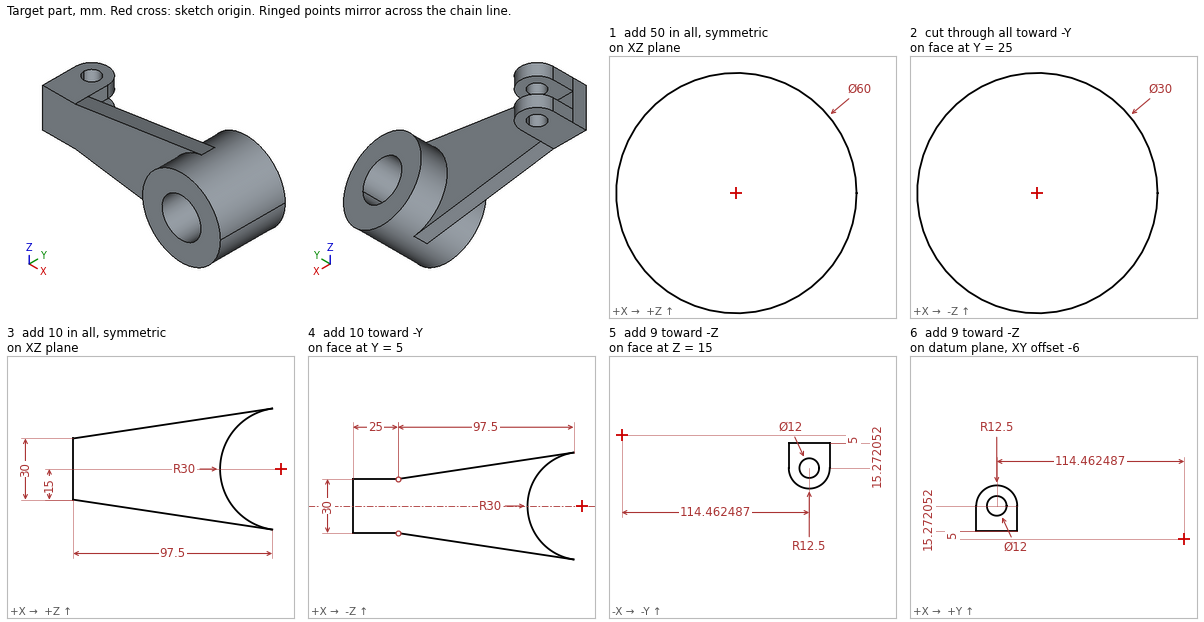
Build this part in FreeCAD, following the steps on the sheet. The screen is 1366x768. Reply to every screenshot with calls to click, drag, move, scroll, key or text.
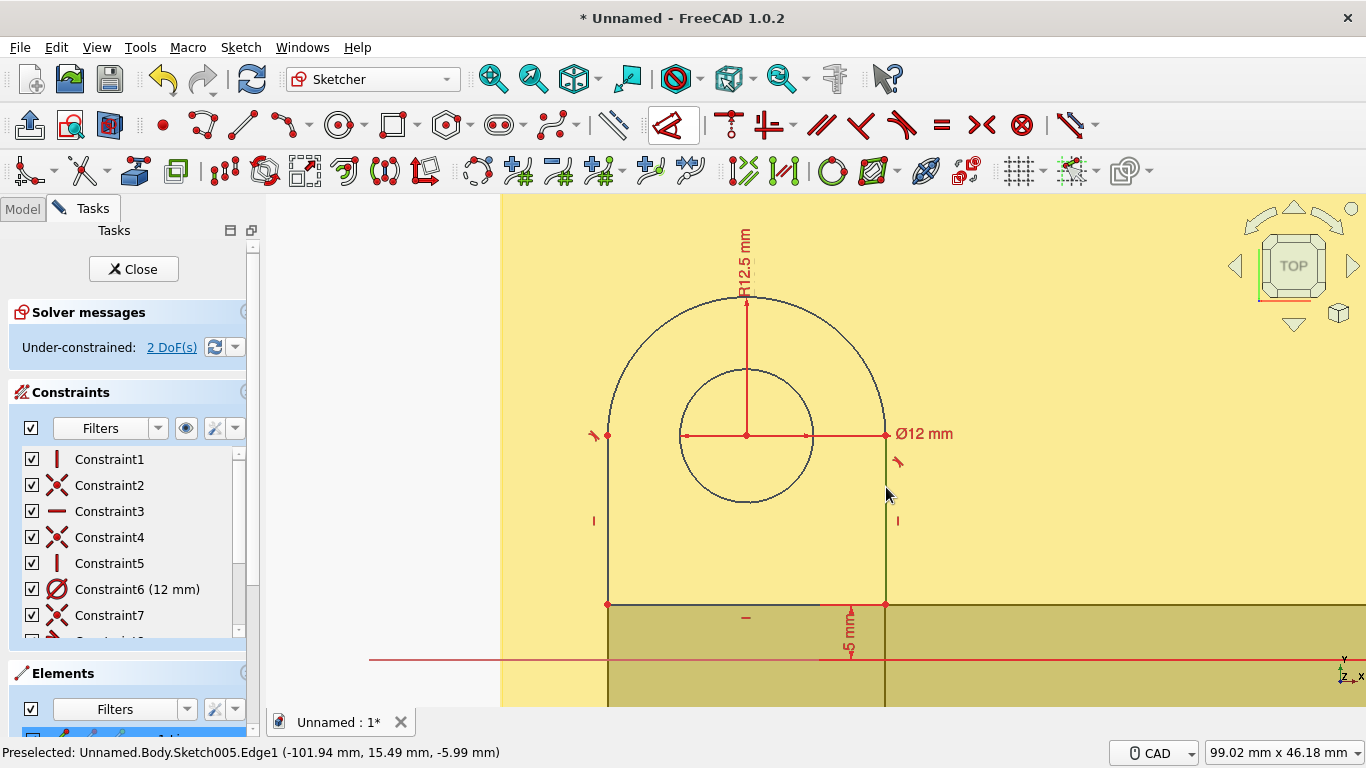
key(i)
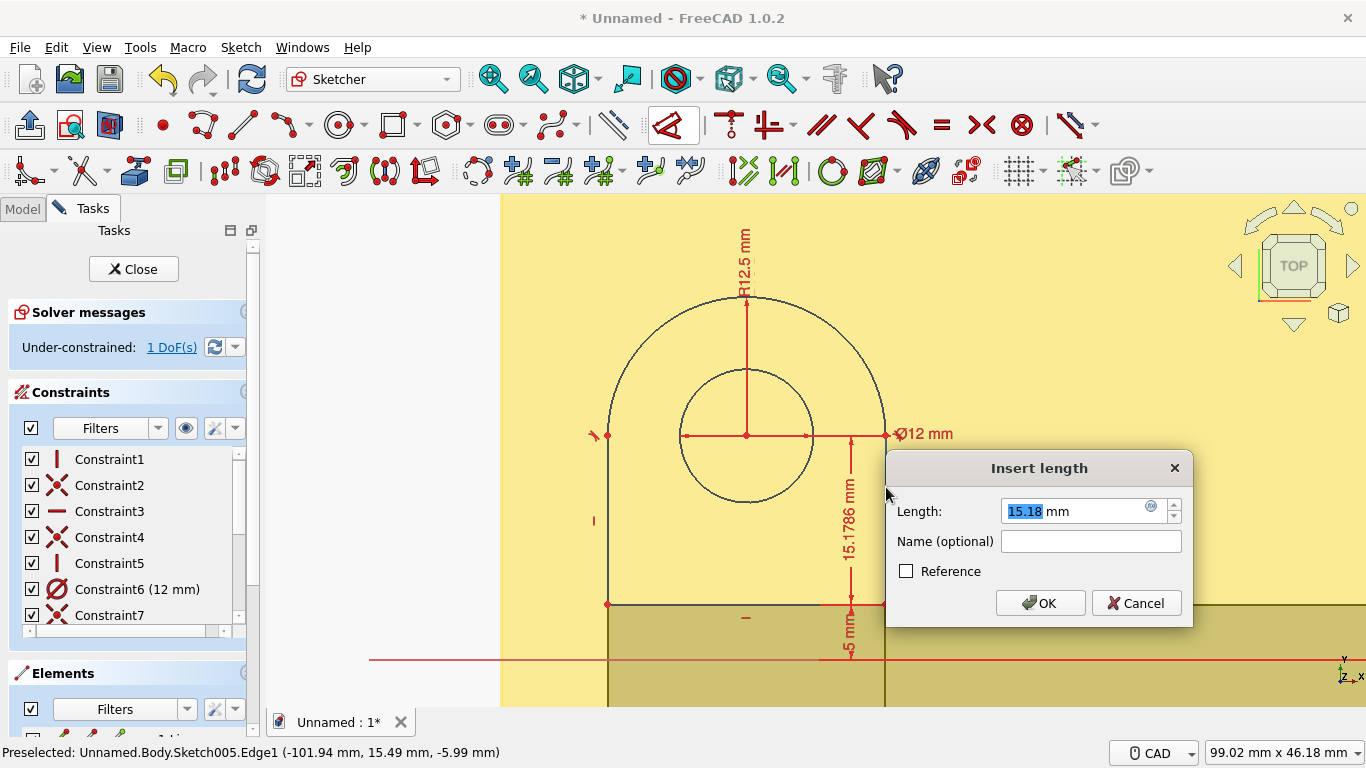
text(15.272052)
key(Return)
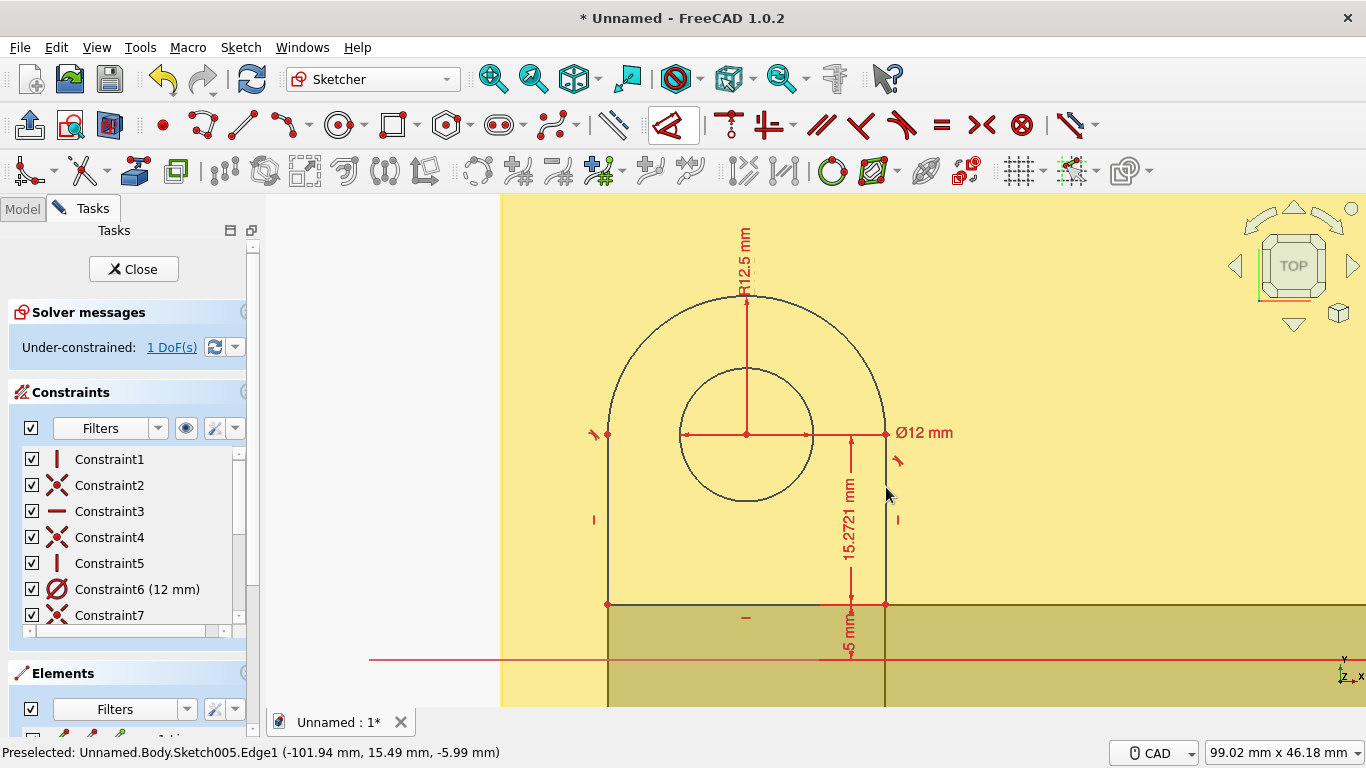
click(747, 435)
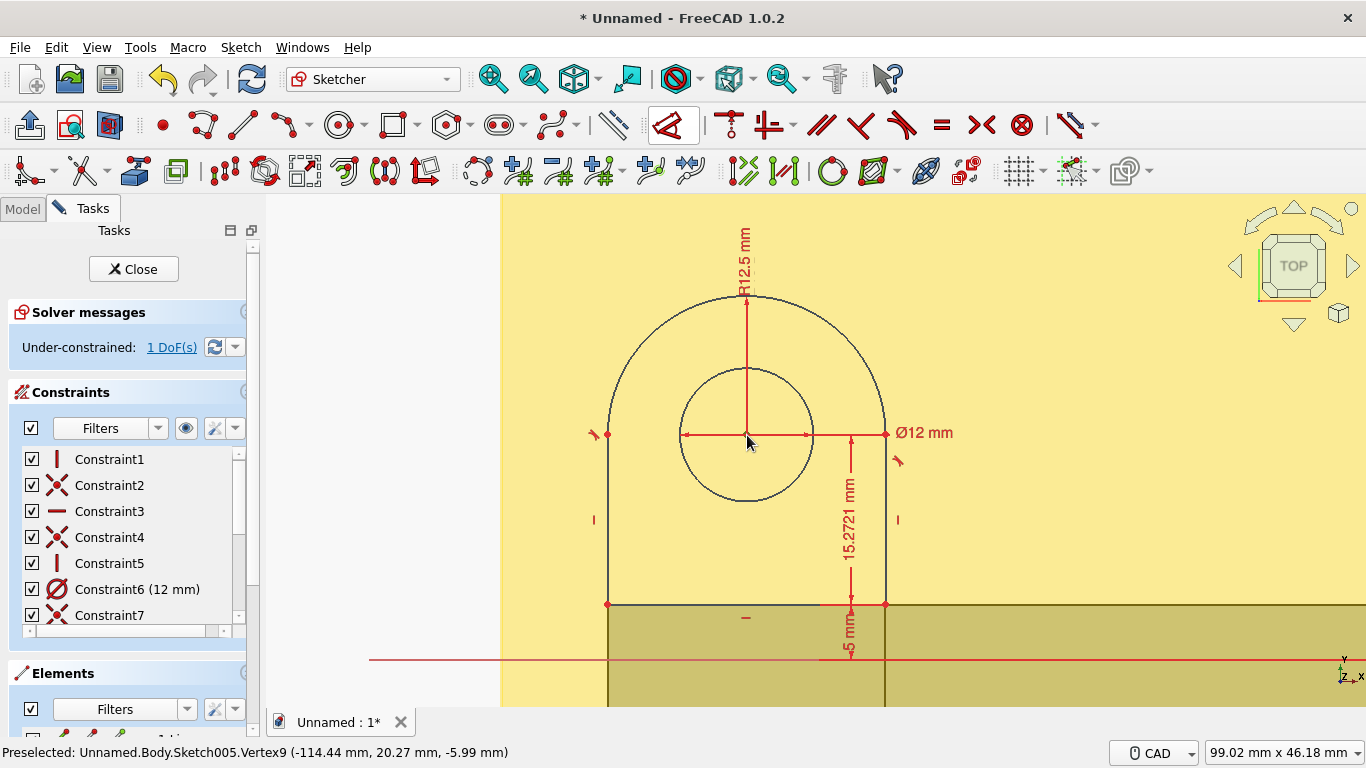
click(694, 126)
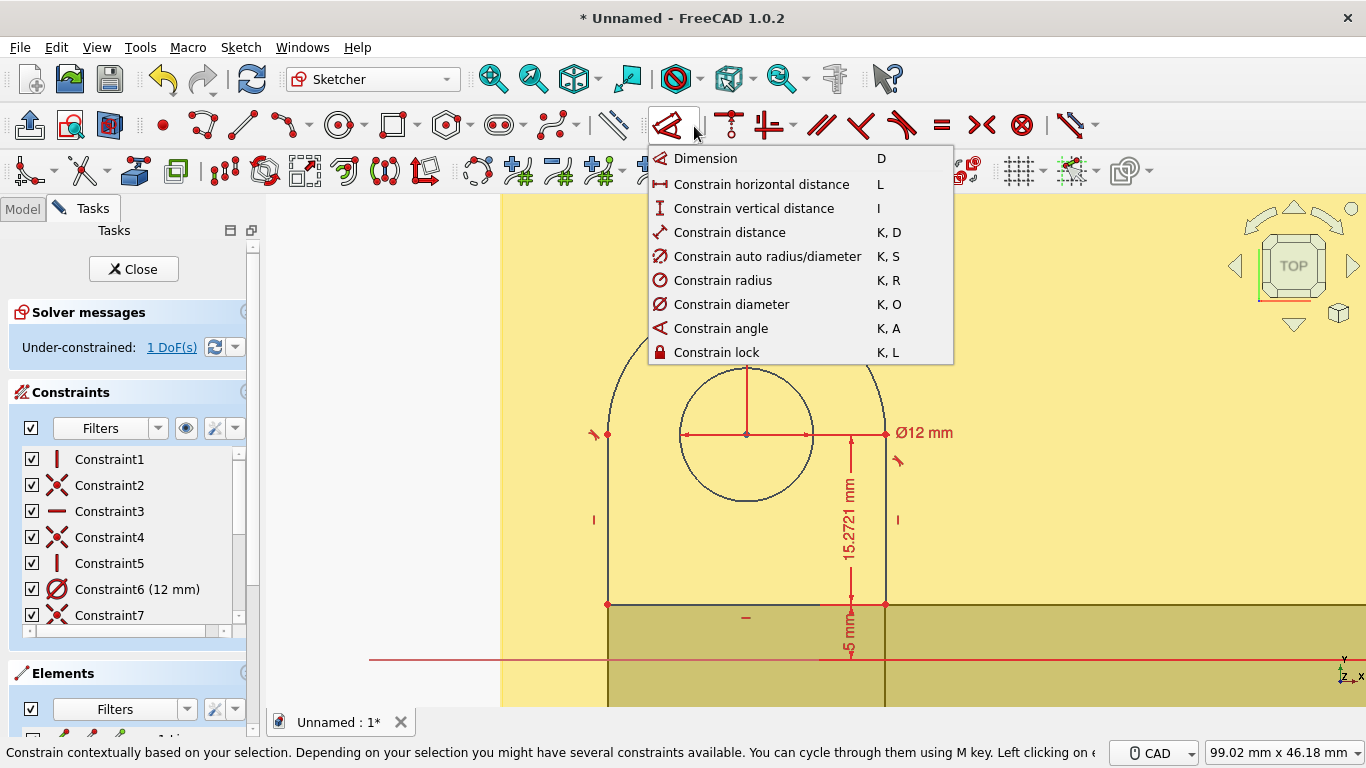
click(801, 184)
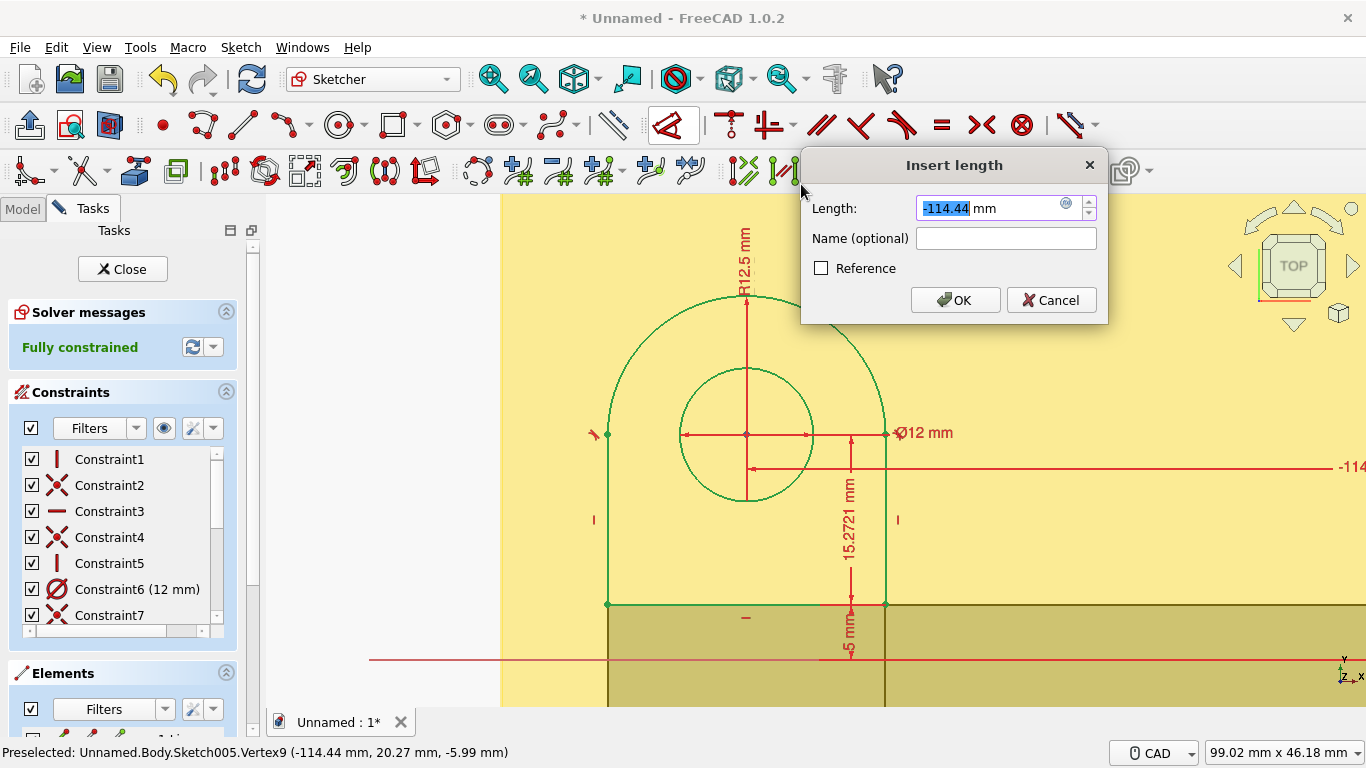
text(-114.462487)
key(Return)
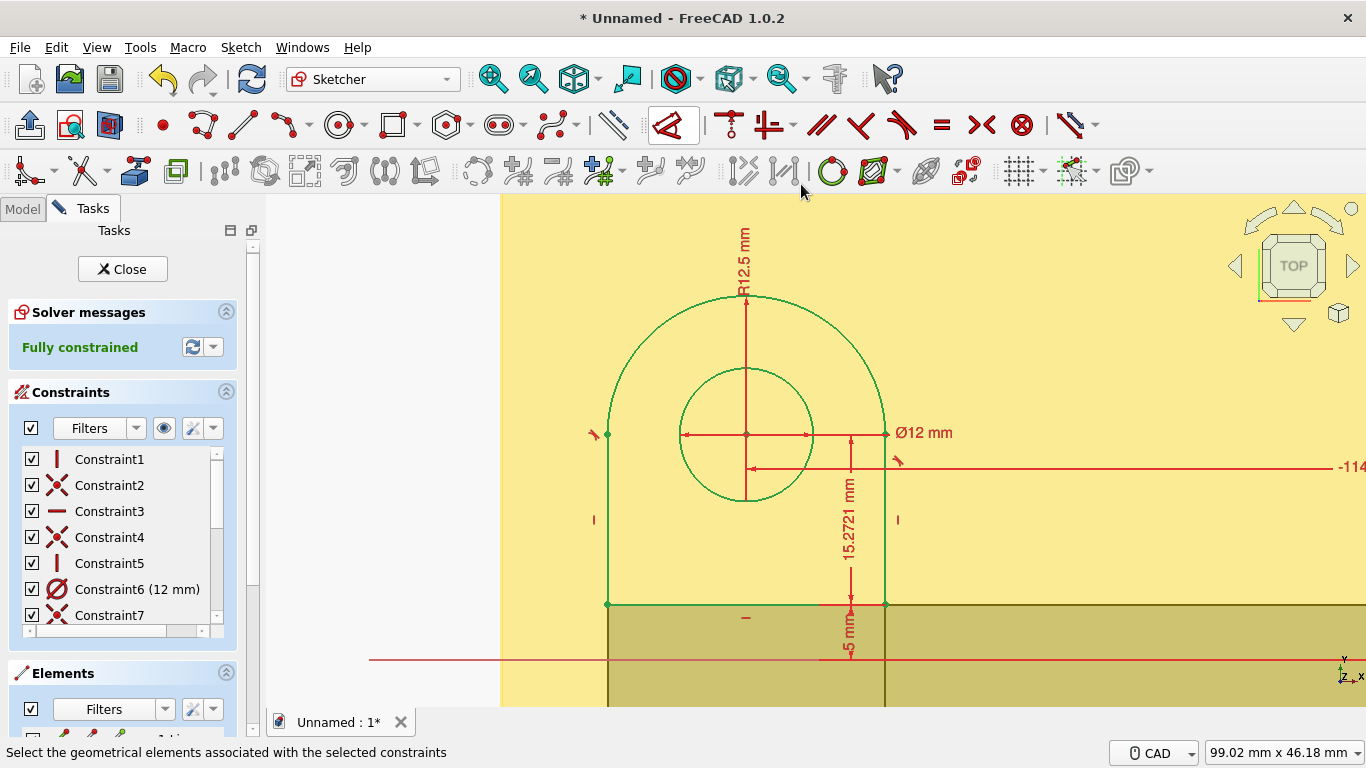
click(123, 269)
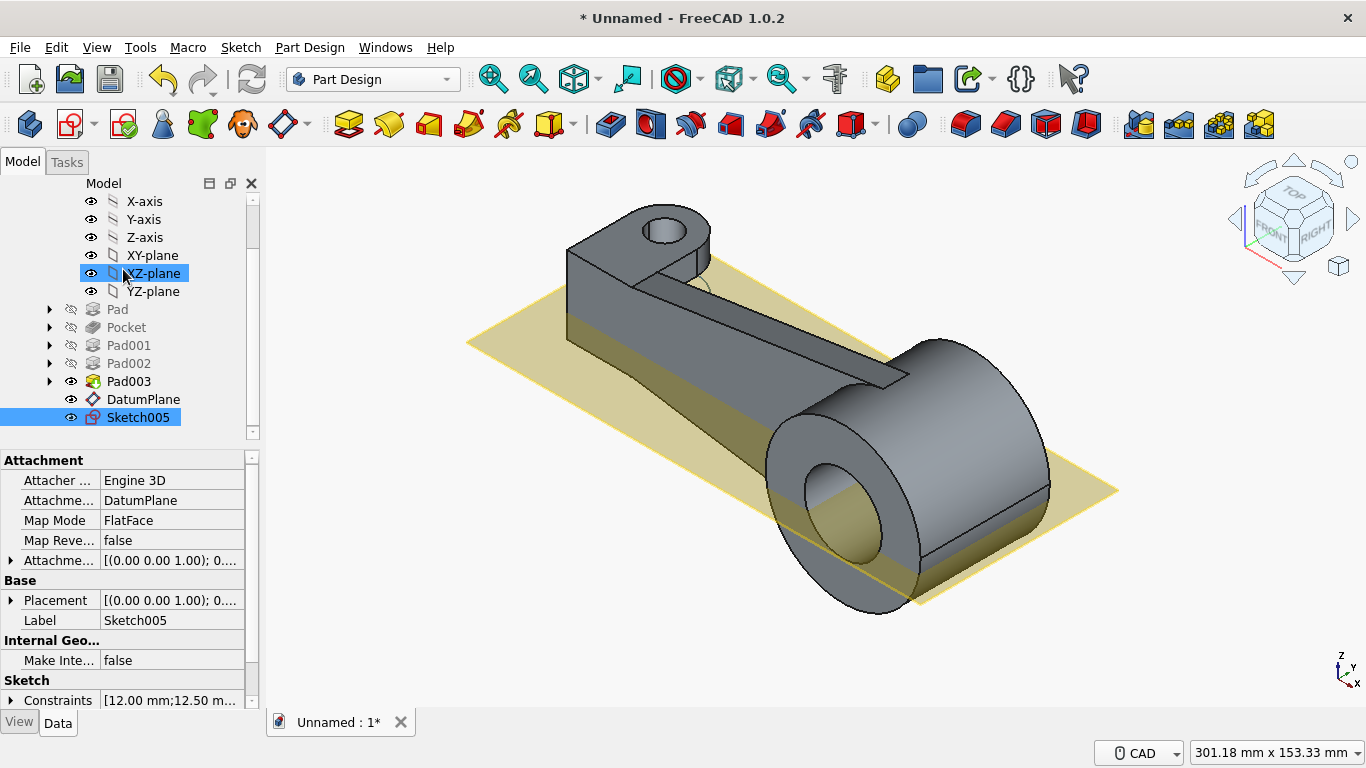
click(350, 124)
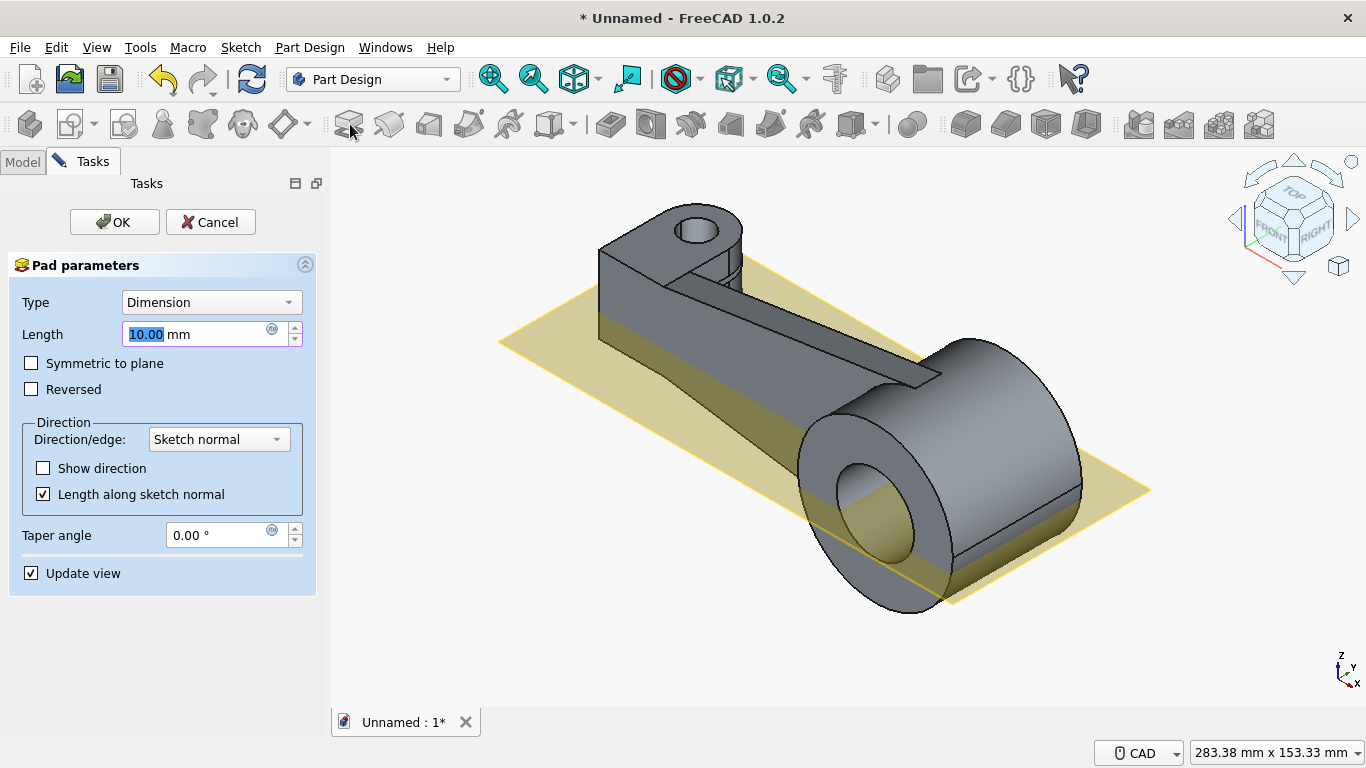
text(9)
key(Tab)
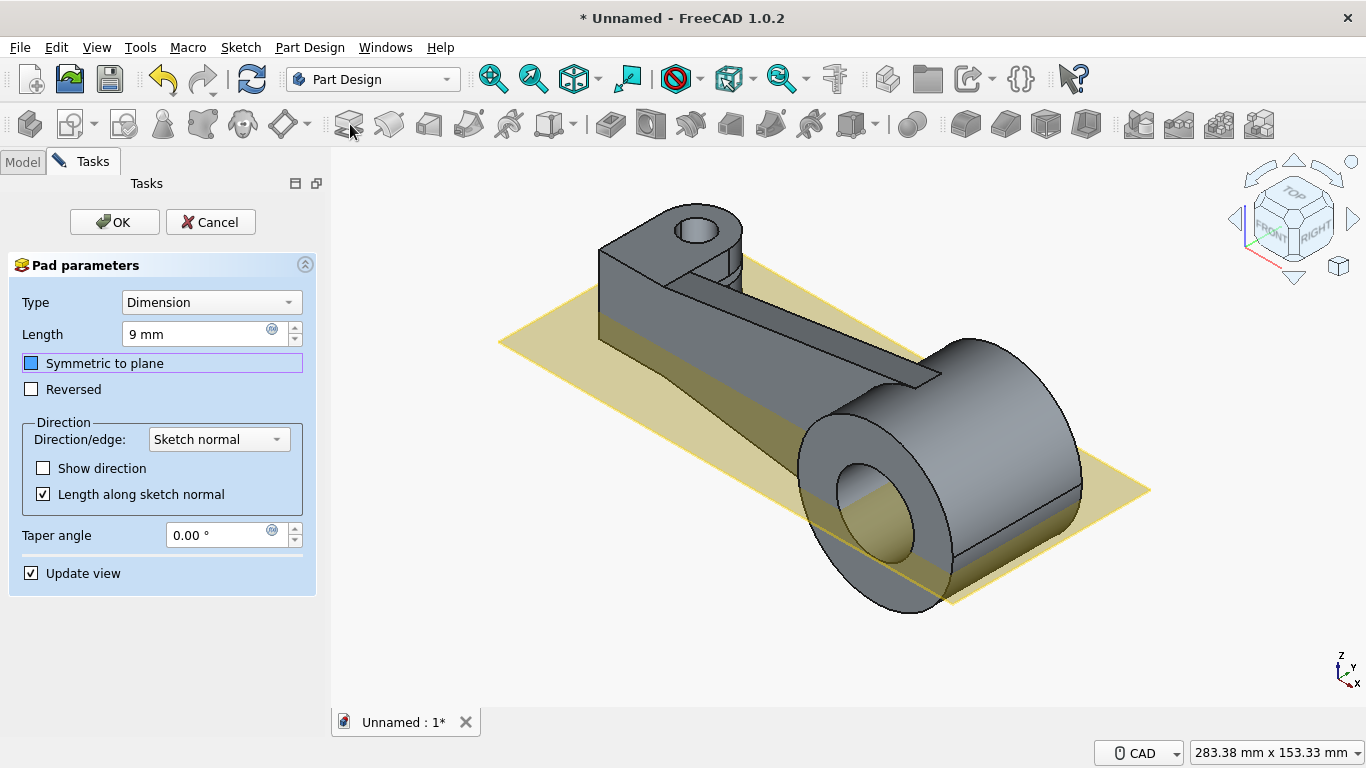
click(30, 389)